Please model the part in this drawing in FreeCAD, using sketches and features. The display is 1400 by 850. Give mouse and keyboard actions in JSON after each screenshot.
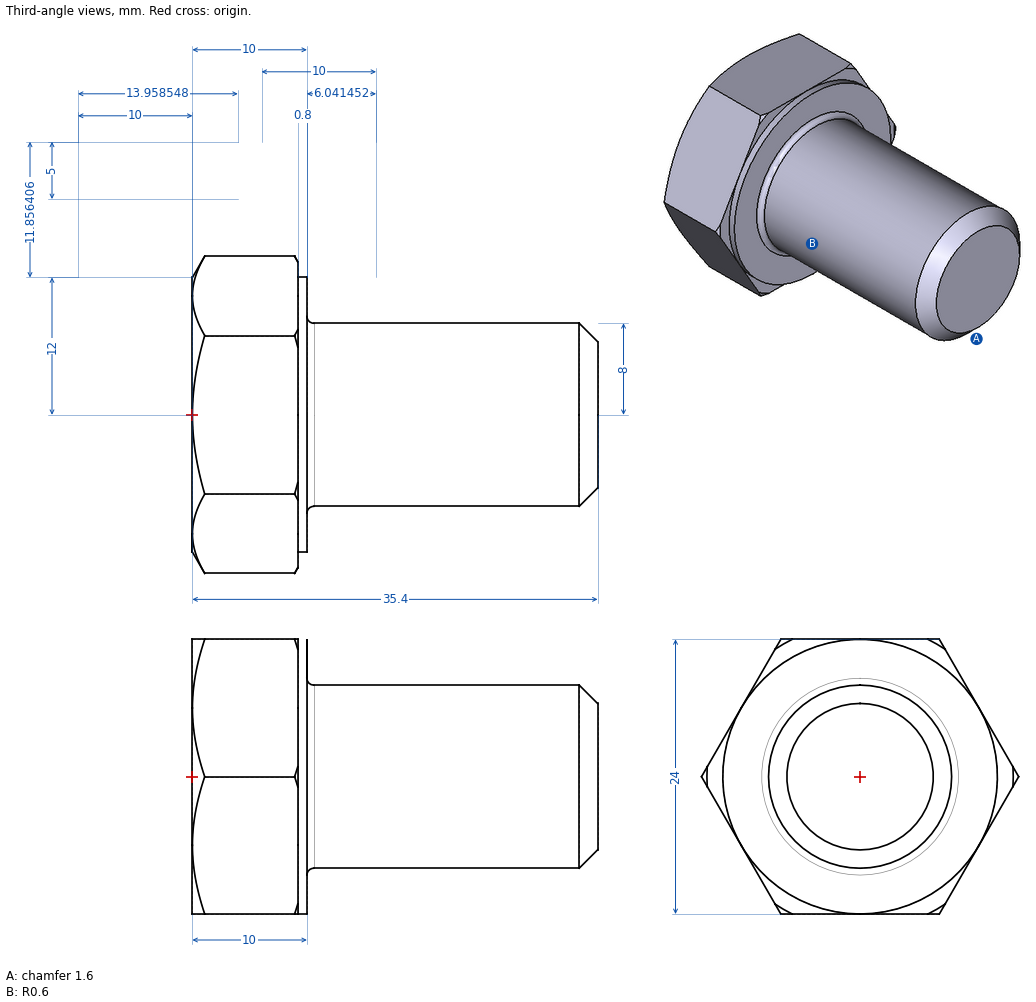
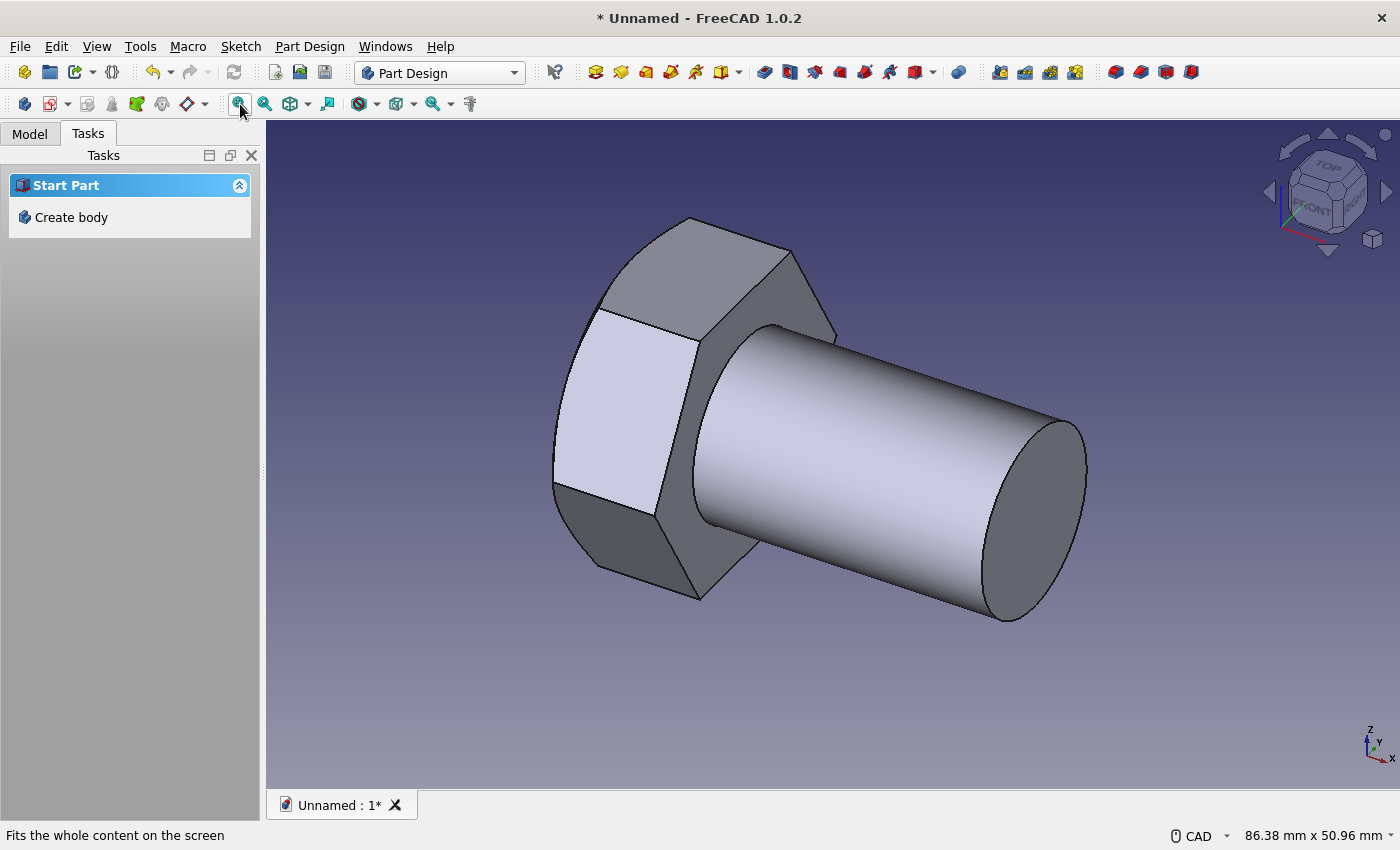
{"action": "left_click", "coordinate": [50, 104]}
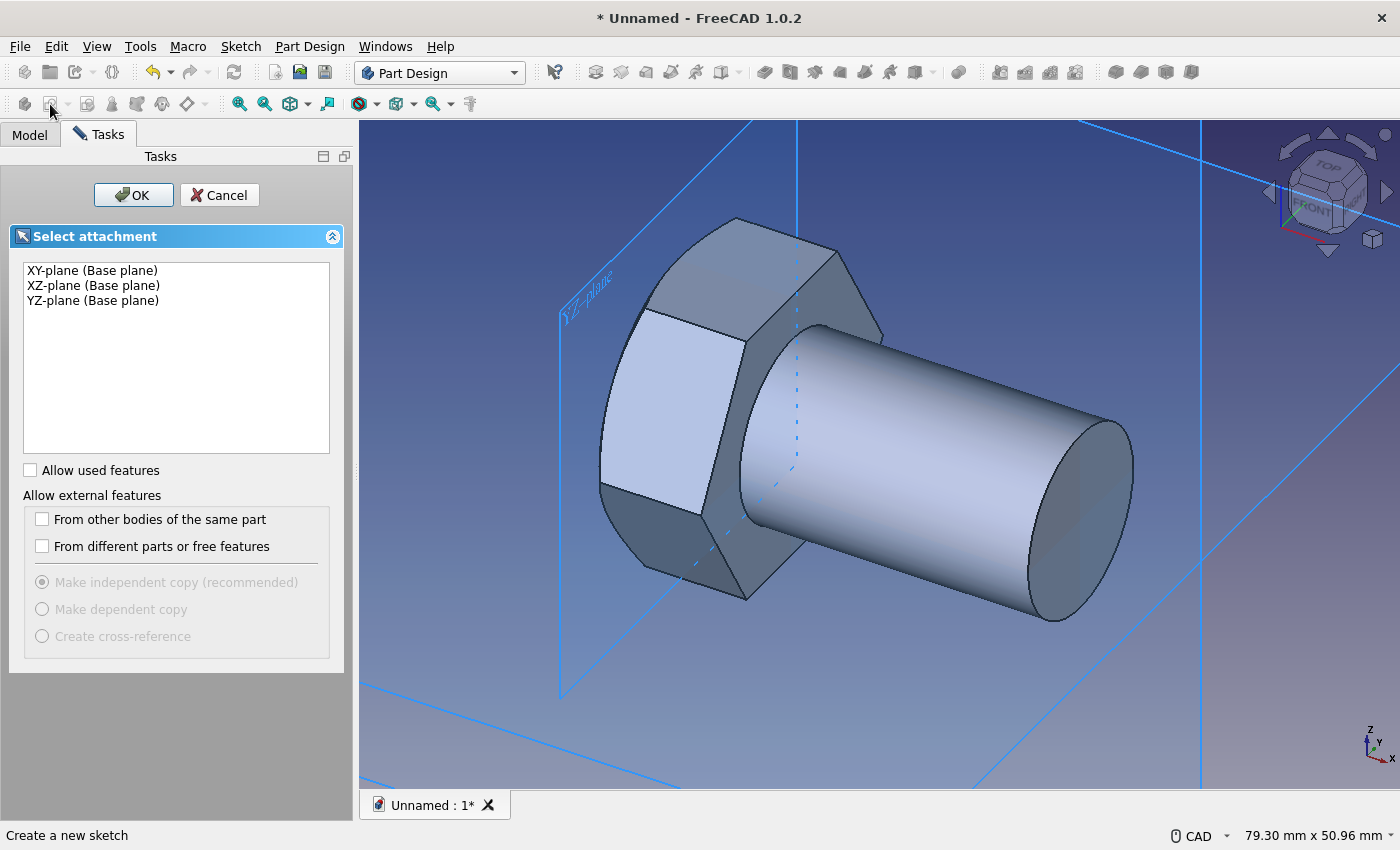
{"action": "left_click", "coordinate": [84, 270]}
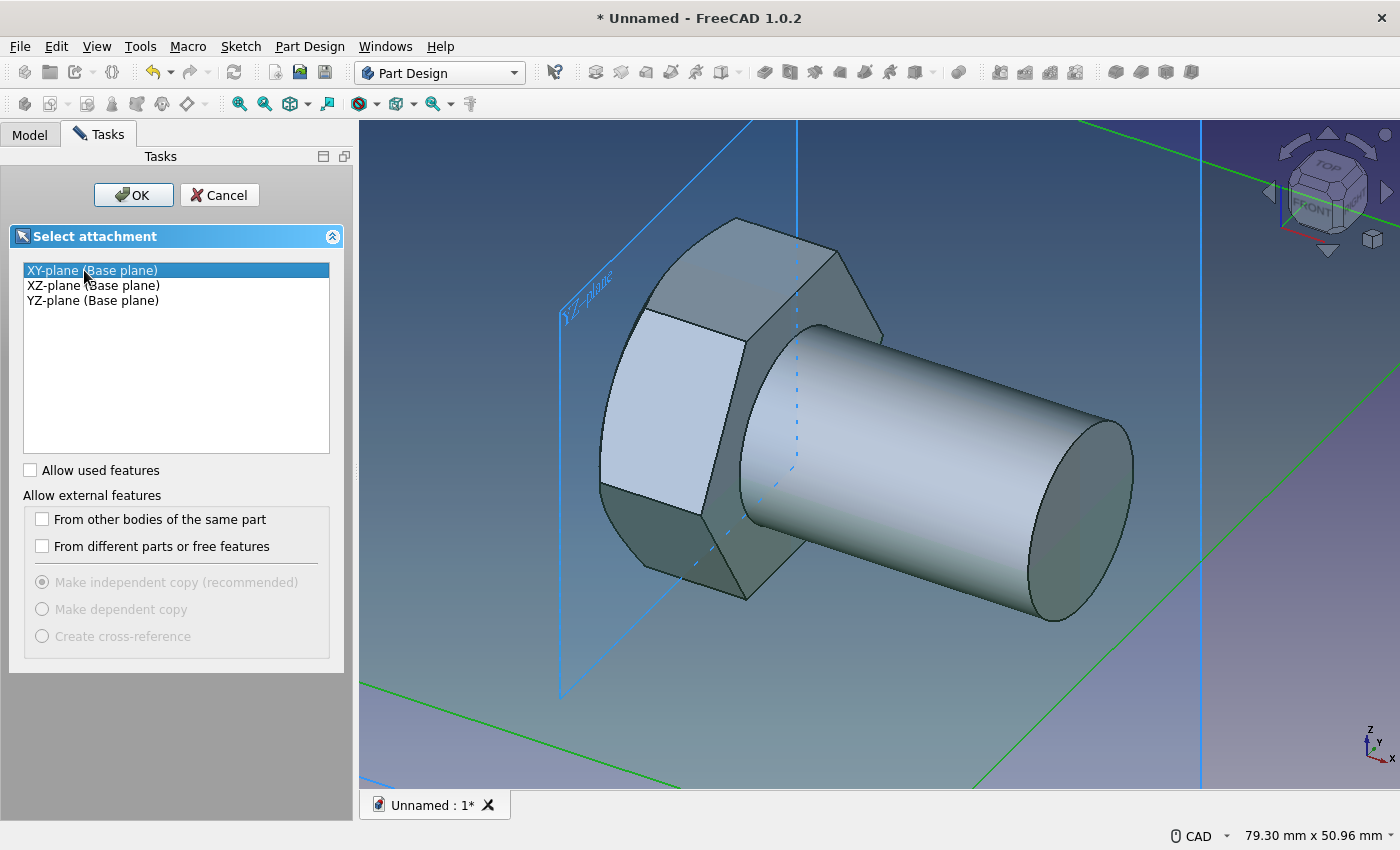
{"action": "left_click", "coordinate": [134, 195]}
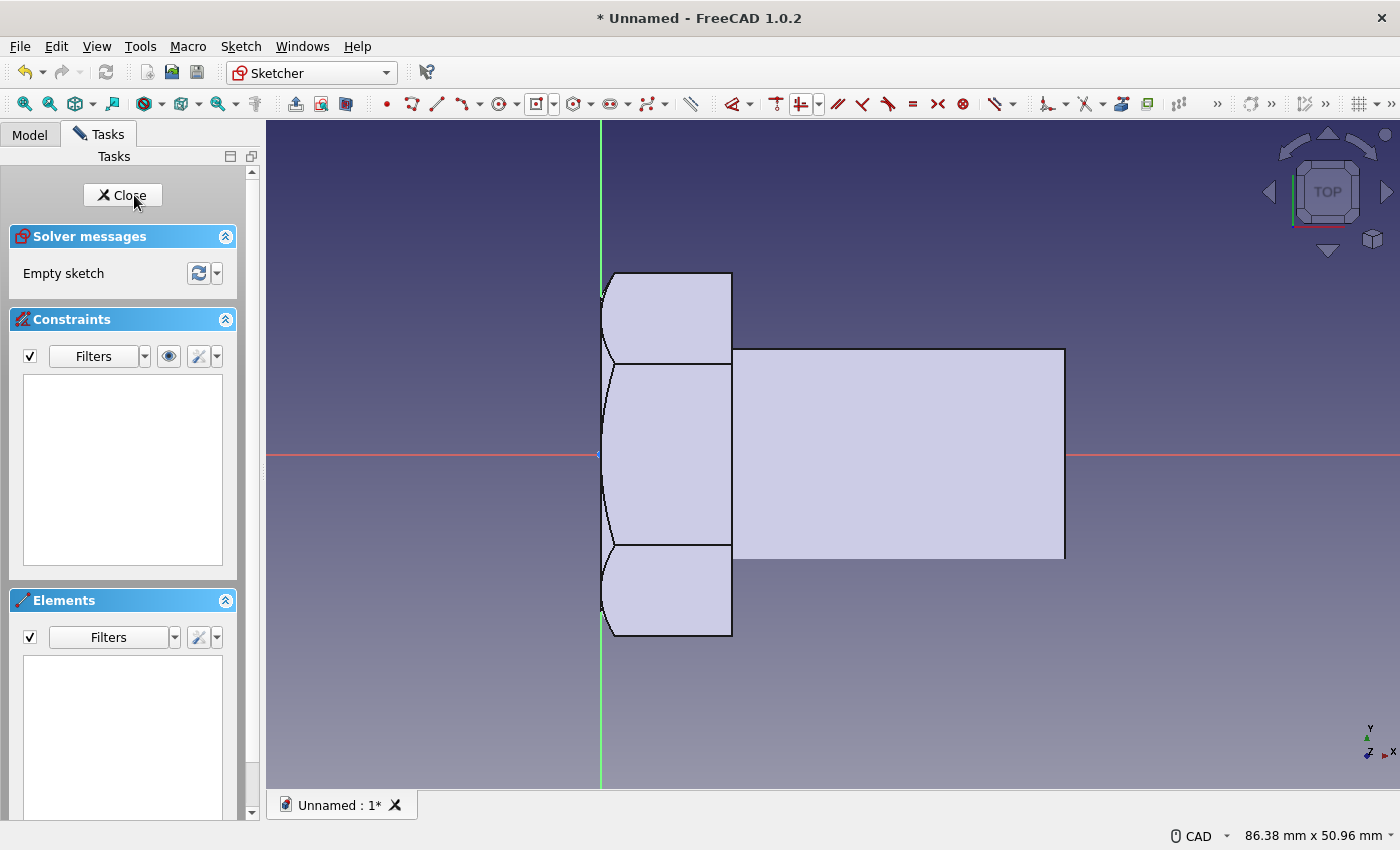
{"action": "key", "text": "q s"}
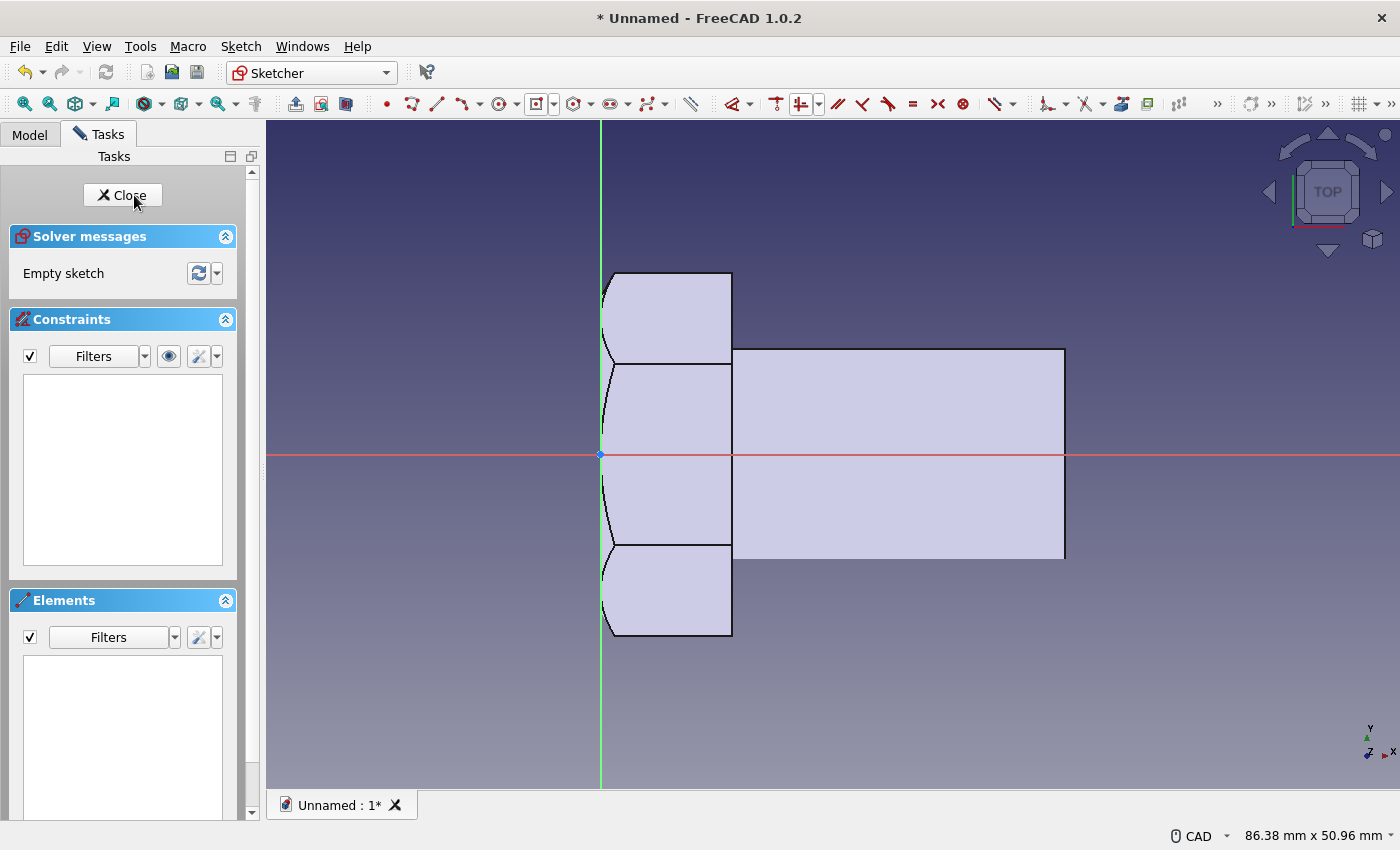
{"action": "scroll", "coordinate": [1029, 761], "scroll_direction": "down", "scroll_amount": 1}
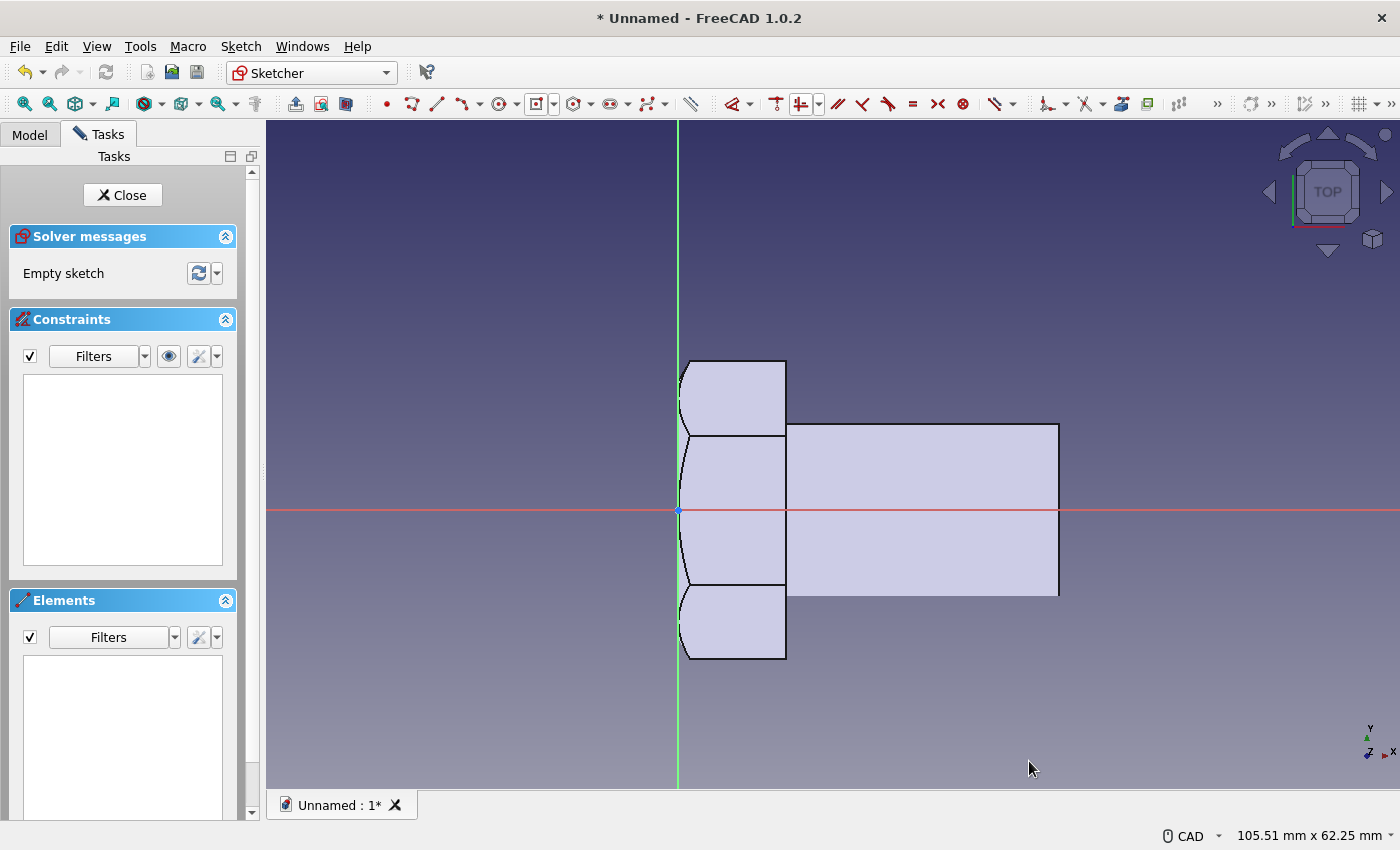
{"action": "scroll", "coordinate": [765, 294], "scroll_direction": "up", "scroll_amount": 3}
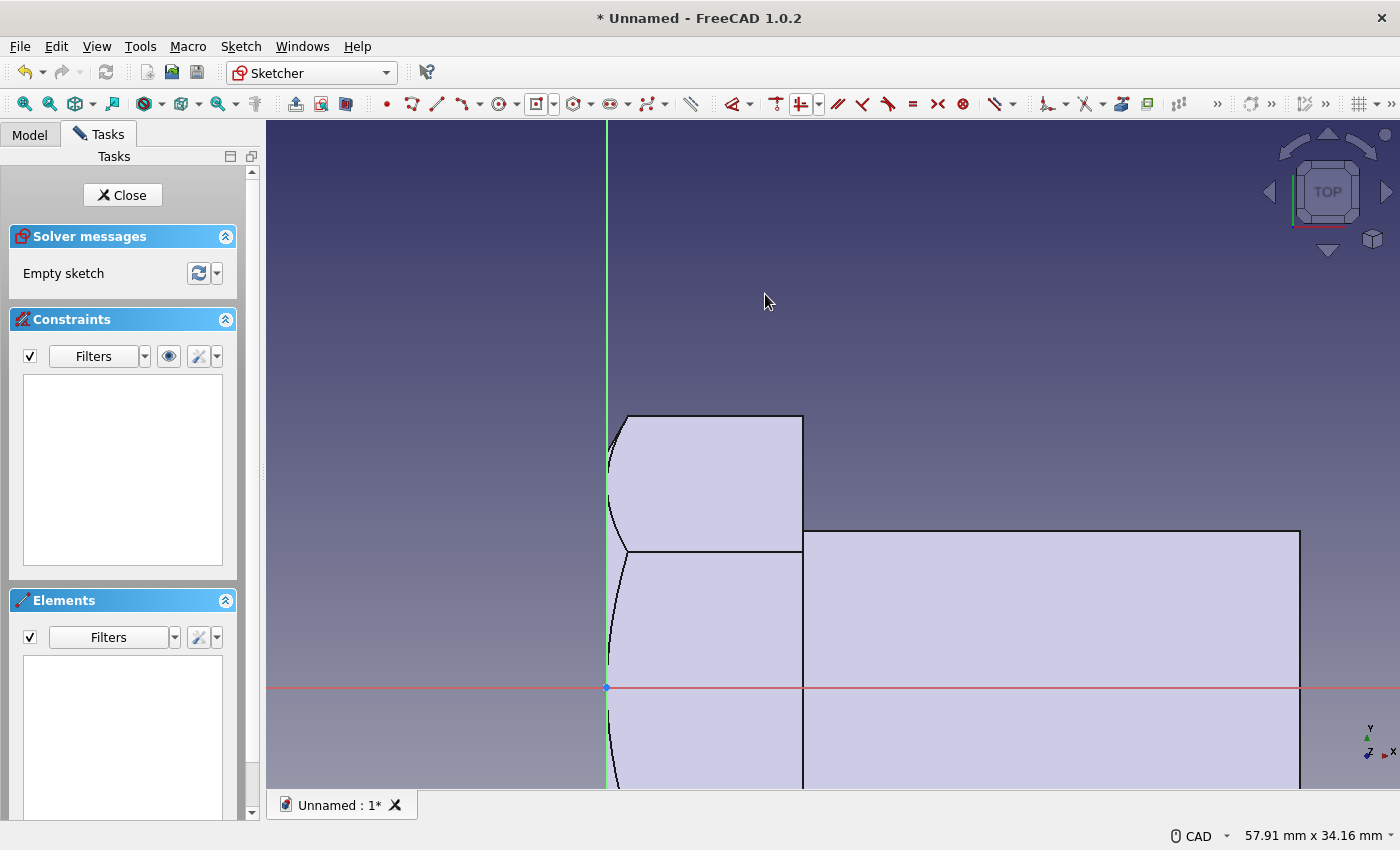
{"action": "key", "text": "g m"}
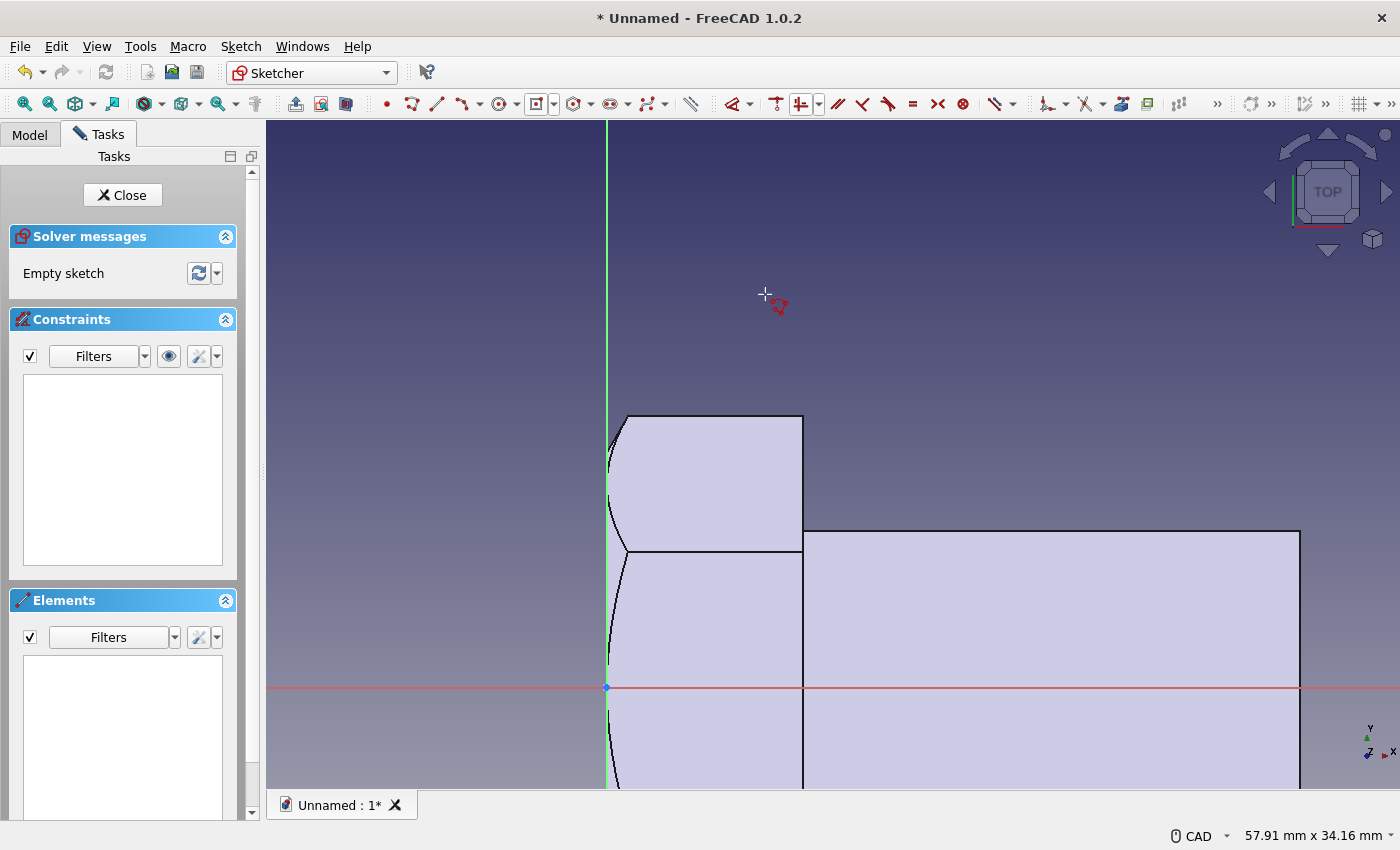
{"action": "left_click", "coordinate": [803, 453]}
{"action": "left_click", "coordinate": [921, 453]}
{"action": "left_click", "coordinate": [921, 221]}
{"action": "left_click", "coordinate": [725, 221]}
{"action": "left_click", "coordinate": [725, 319]}
{"action": "left_click", "coordinate": [803, 454]}
{"action": "key", "text": "Escape"}
{"action": "key", "text": "Escape"}